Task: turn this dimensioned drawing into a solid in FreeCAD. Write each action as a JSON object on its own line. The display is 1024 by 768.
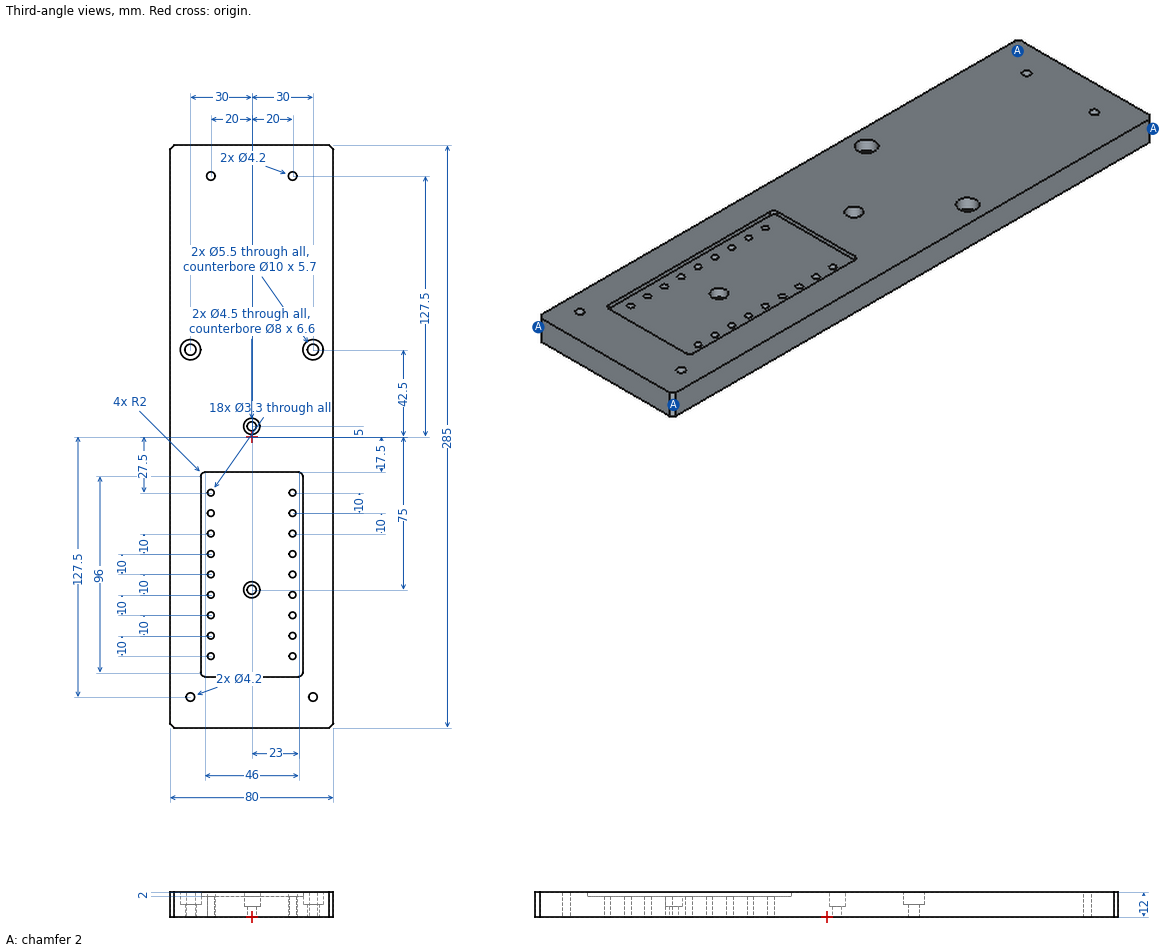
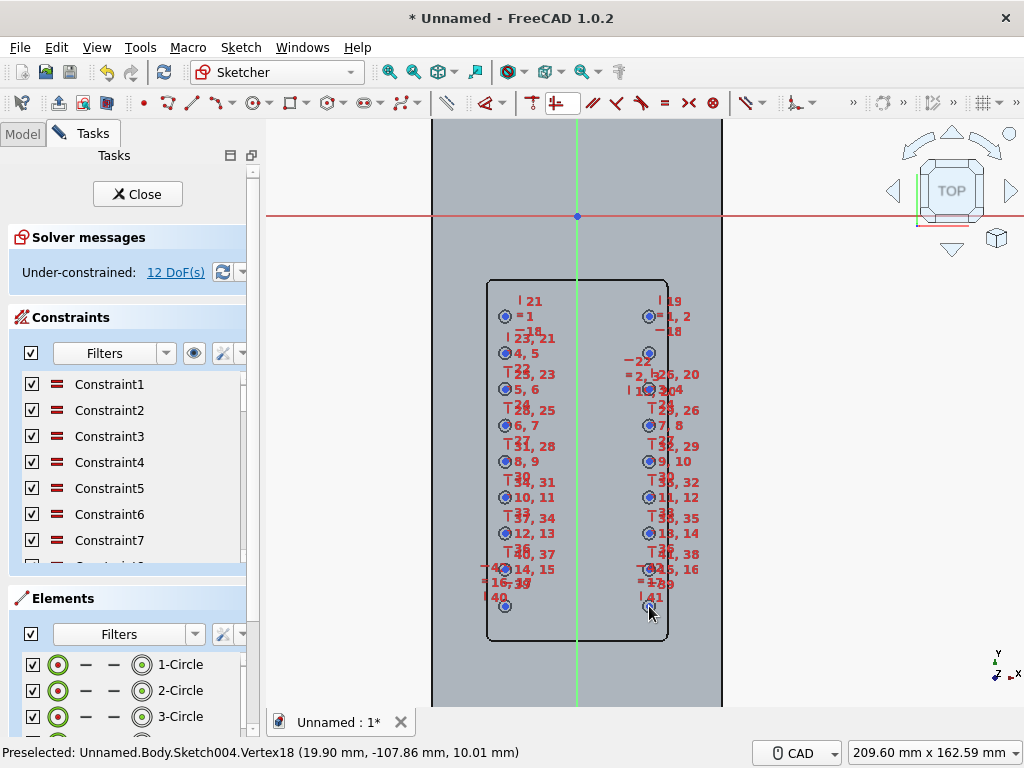
{"action": "key", "text": "d"}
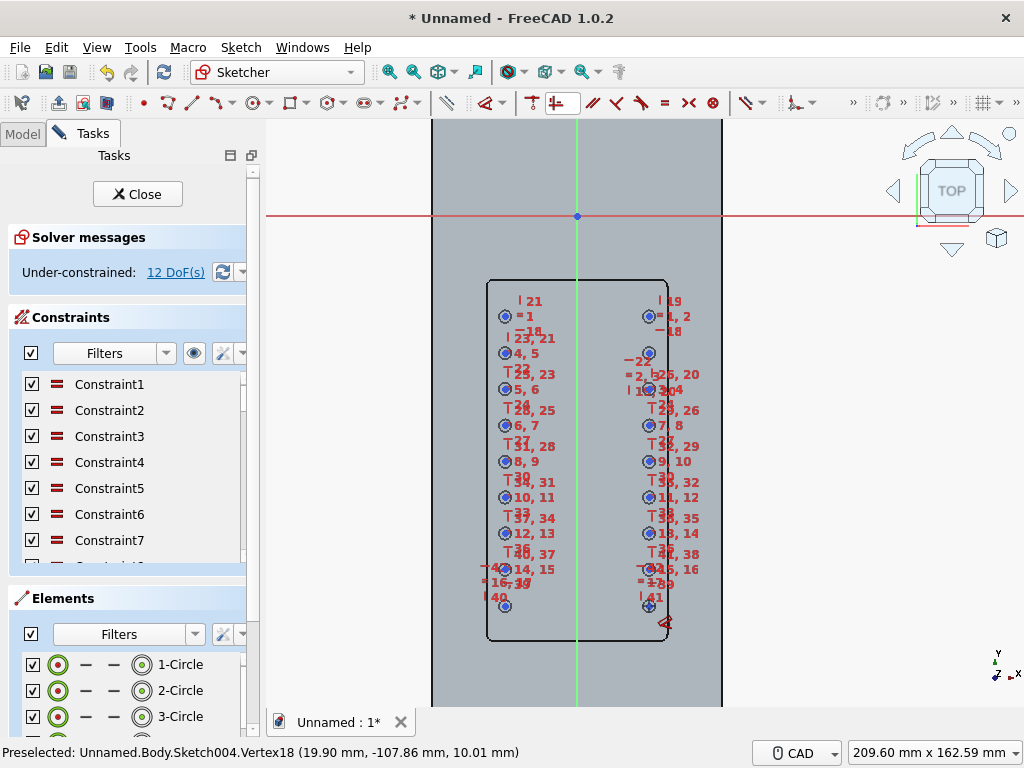
{"action": "scroll", "coordinate": [505, 310], "scroll_direction": "up", "scroll_amount": 7}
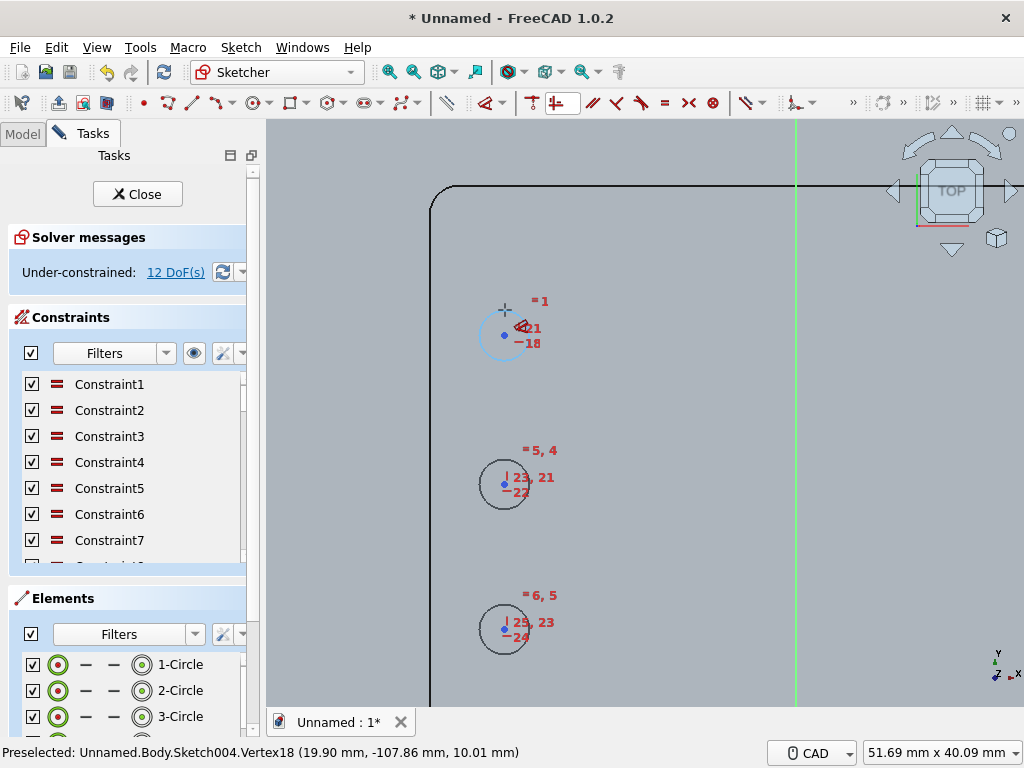
{"action": "left_click", "coordinate": [505, 311]}
{"action": "left_click", "coordinate": [506, 279]}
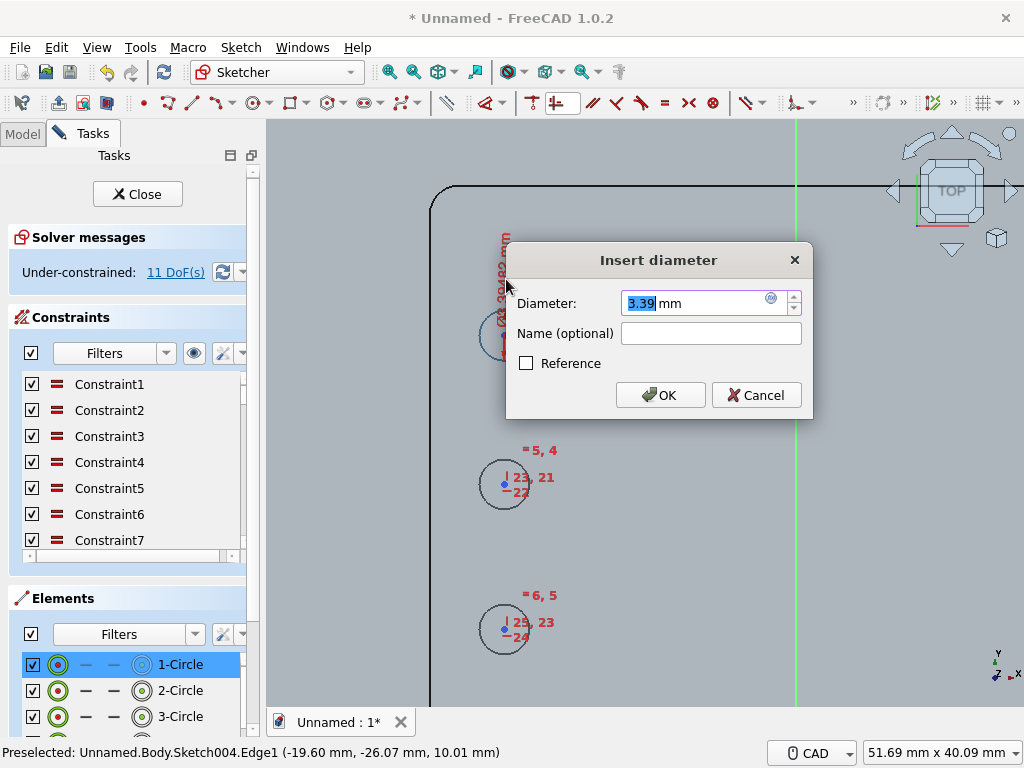
{"action": "type", "text": "3.3"}
{"action": "key", "text": "Return"}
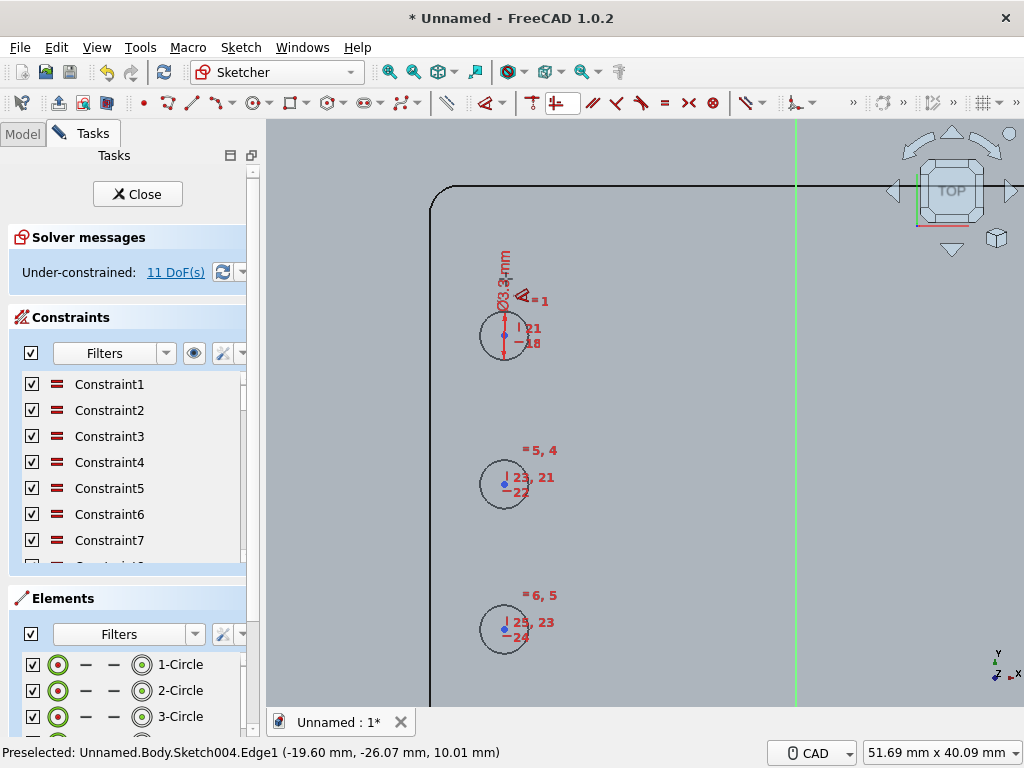
{"action": "scroll", "coordinate": [505, 309], "scroll_direction": "down", "scroll_amount": 7}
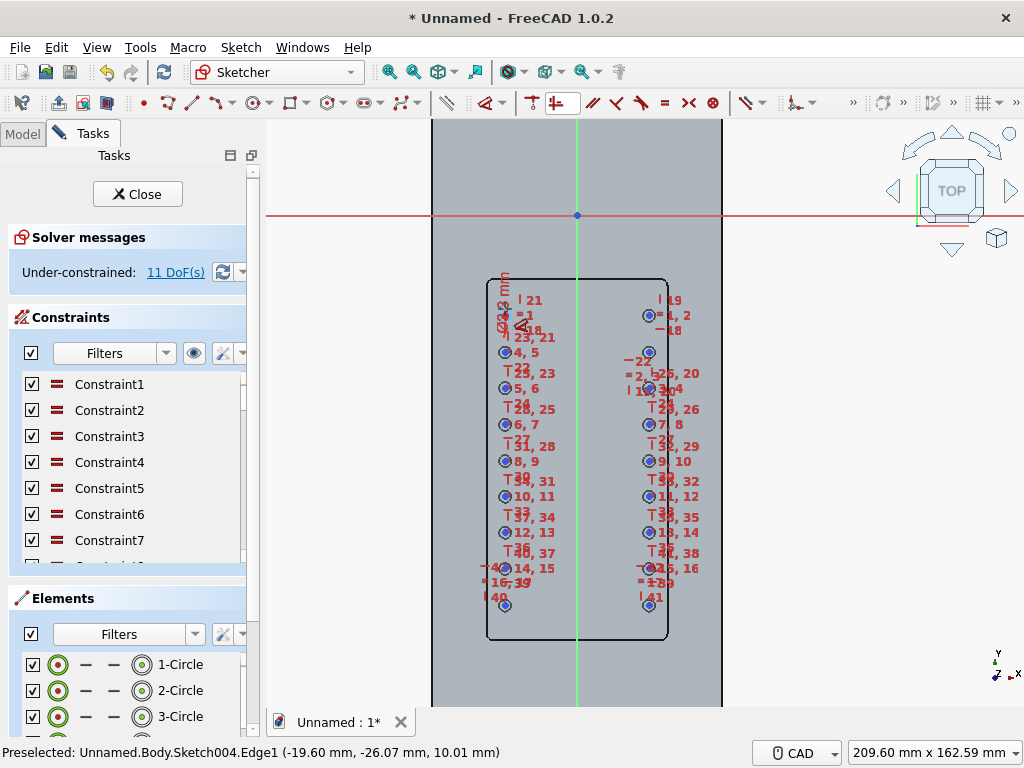
{"action": "left_click", "coordinate": [505, 316]}
{"action": "left_click", "coordinate": [541, 182]}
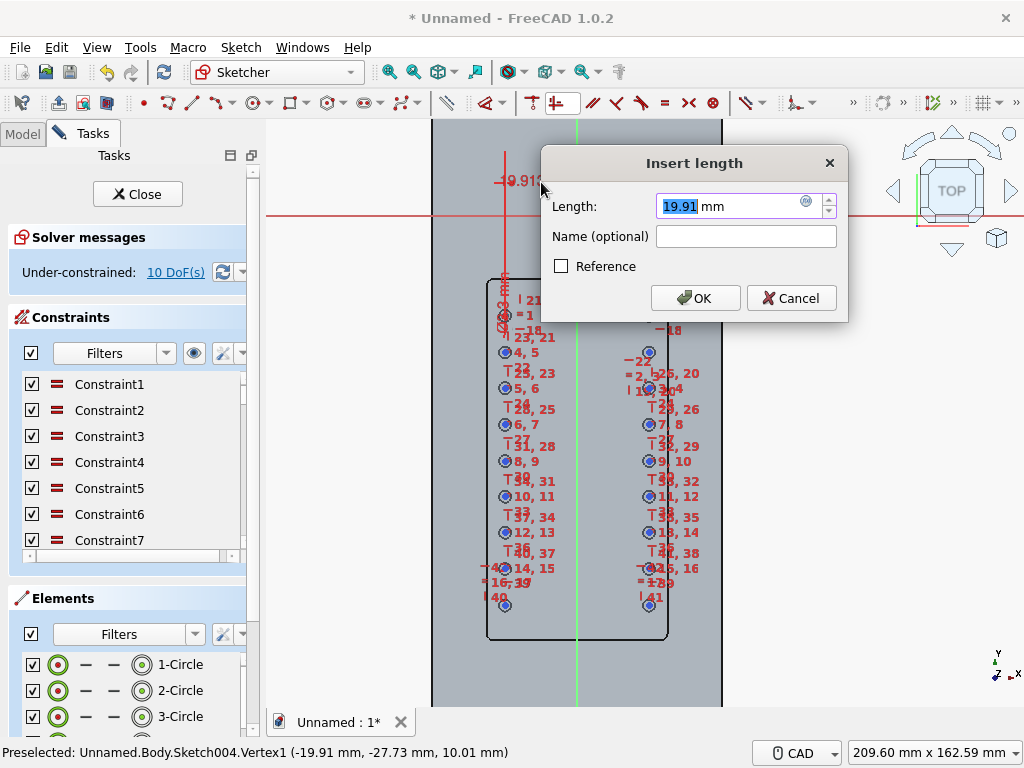
{"action": "type", "text": "20"}
{"action": "key", "text": "Return"}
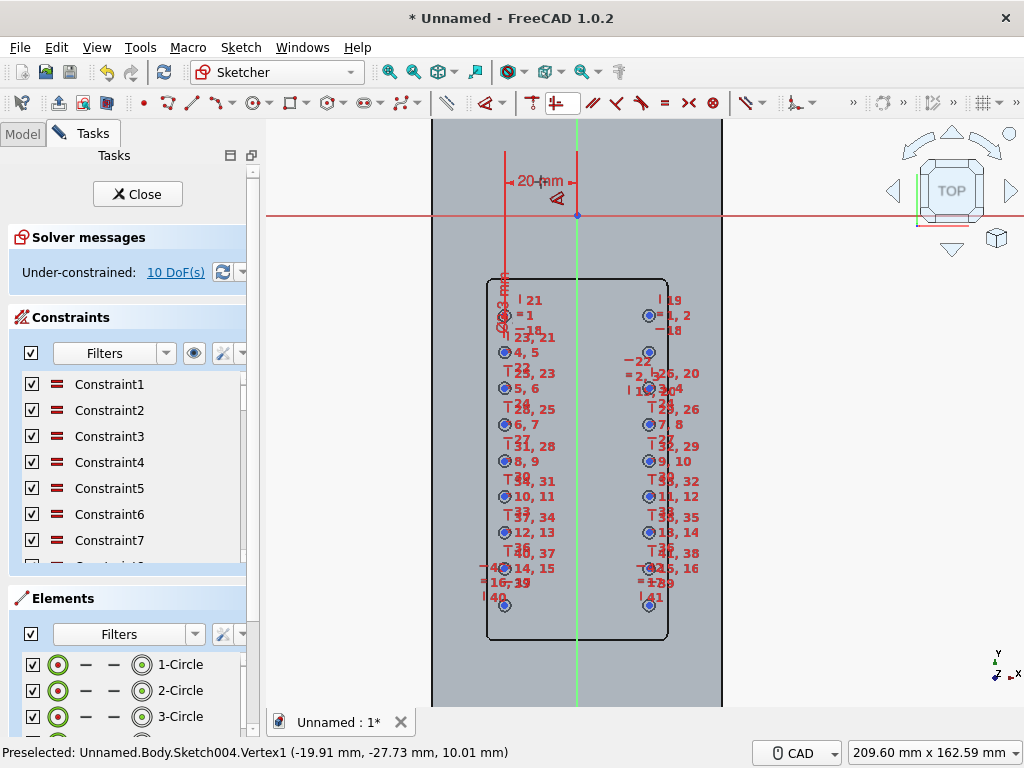
{"action": "left_click", "coordinate": [649, 316]}
{"action": "left_click", "coordinate": [613, 182]}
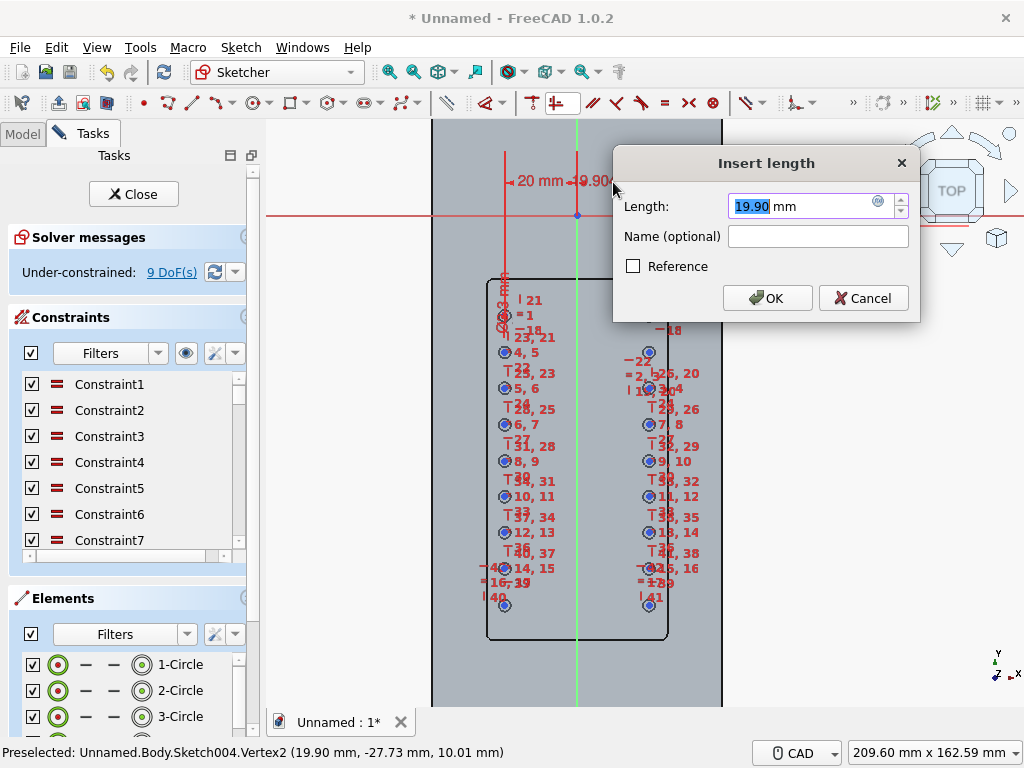
{"action": "type", "text": "20"}
{"action": "key", "text": "Return"}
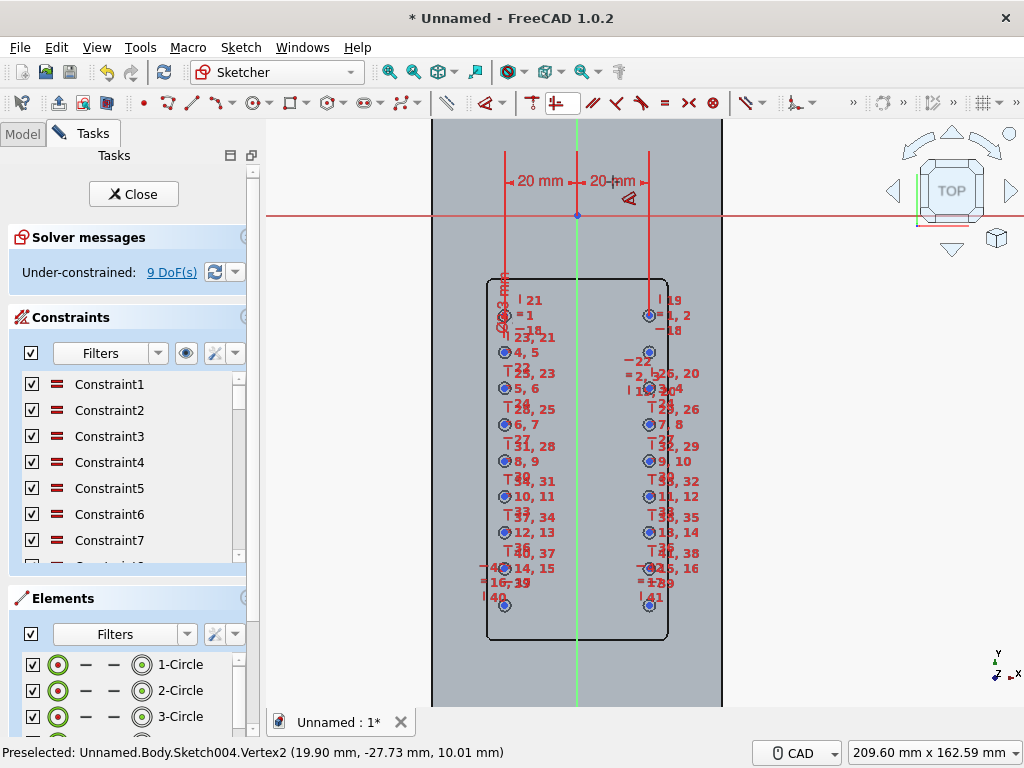
{"action": "left_click", "coordinate": [649, 316]}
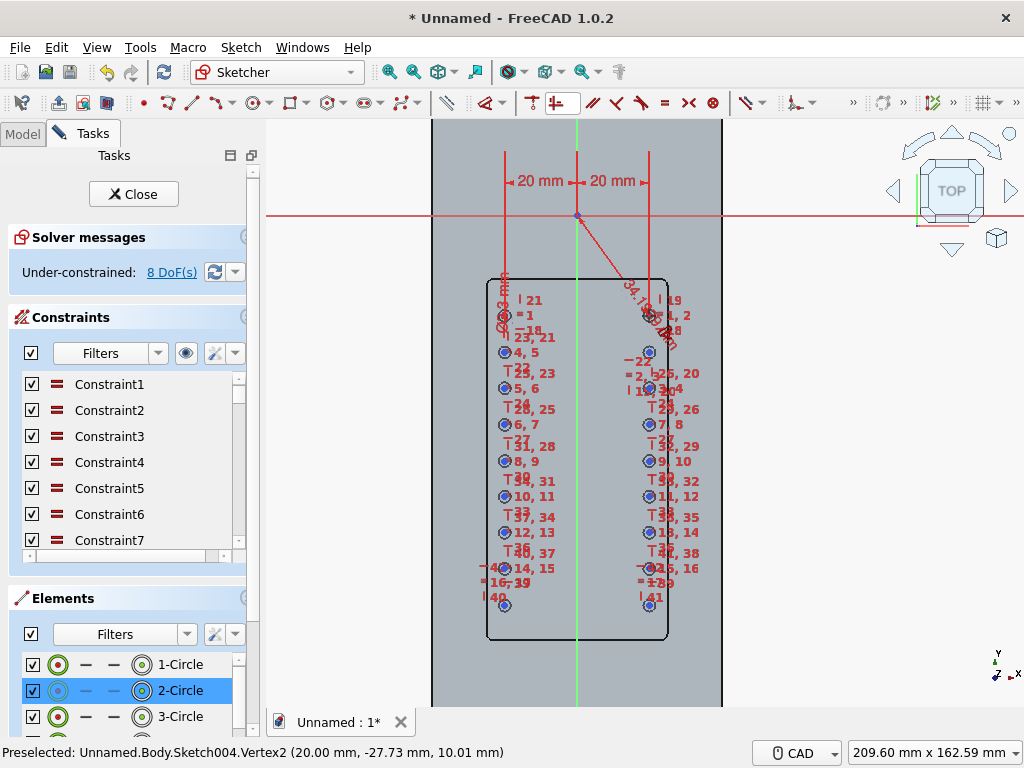
{"action": "left_click", "coordinate": [649, 352]}
{"action": "left_click", "coordinate": [683, 334]}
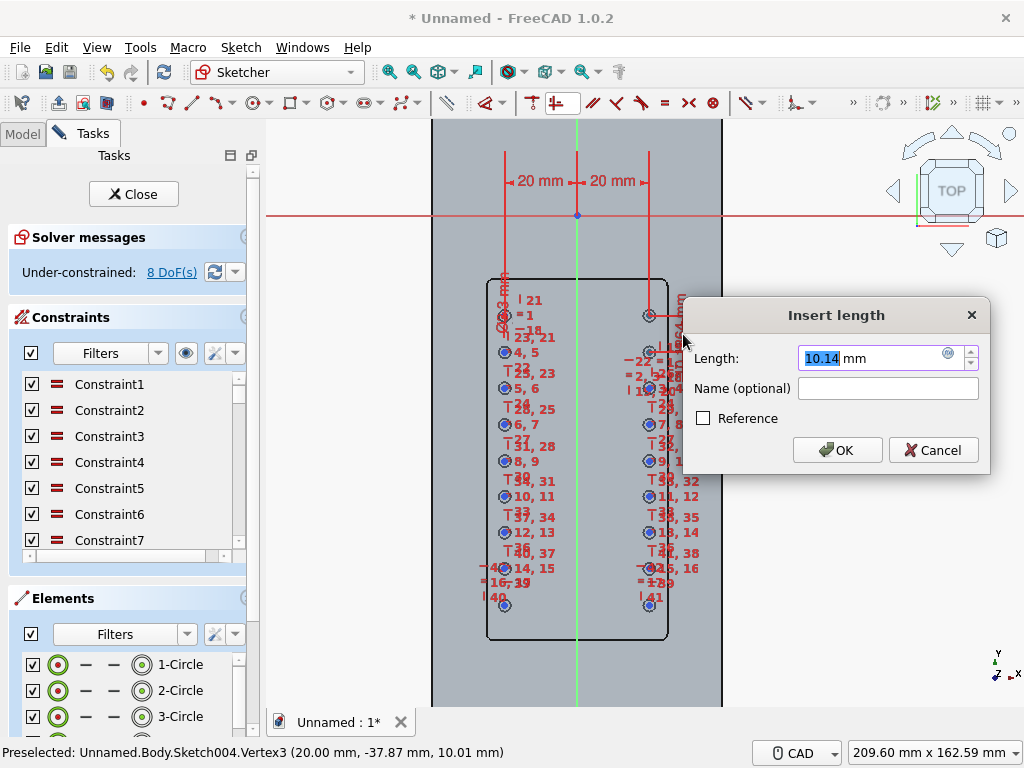
{"action": "type", "text": "10"}
{"action": "key", "text": "Return"}